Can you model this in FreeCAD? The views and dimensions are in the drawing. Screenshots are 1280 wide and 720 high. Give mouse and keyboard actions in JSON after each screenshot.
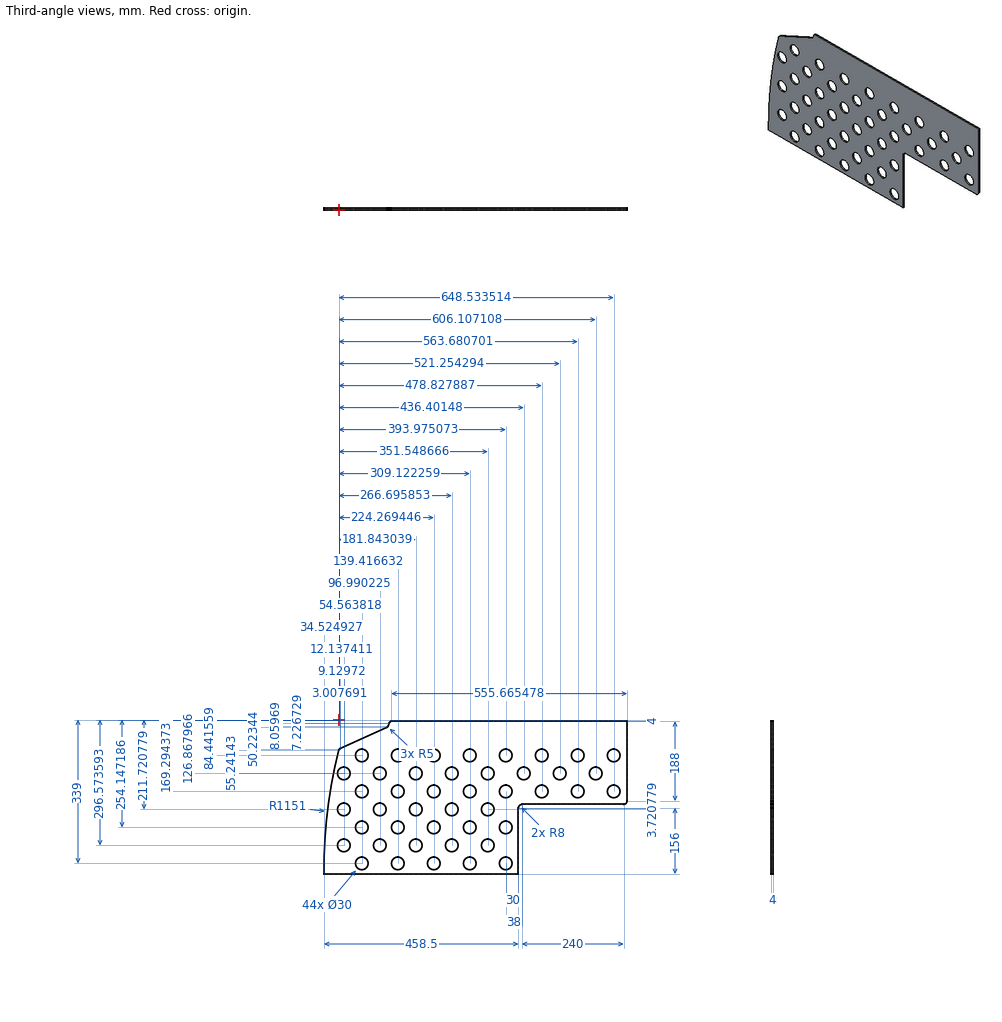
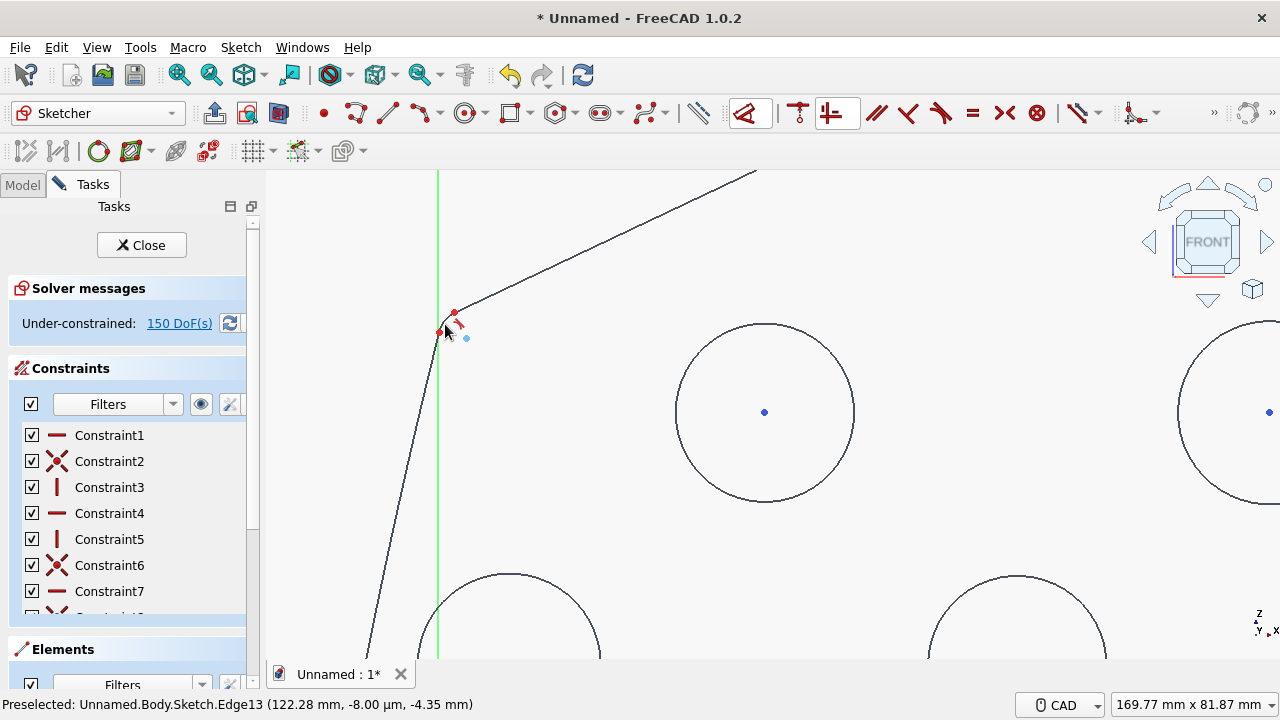
{"action": "left_click", "coordinate": [439, 326]}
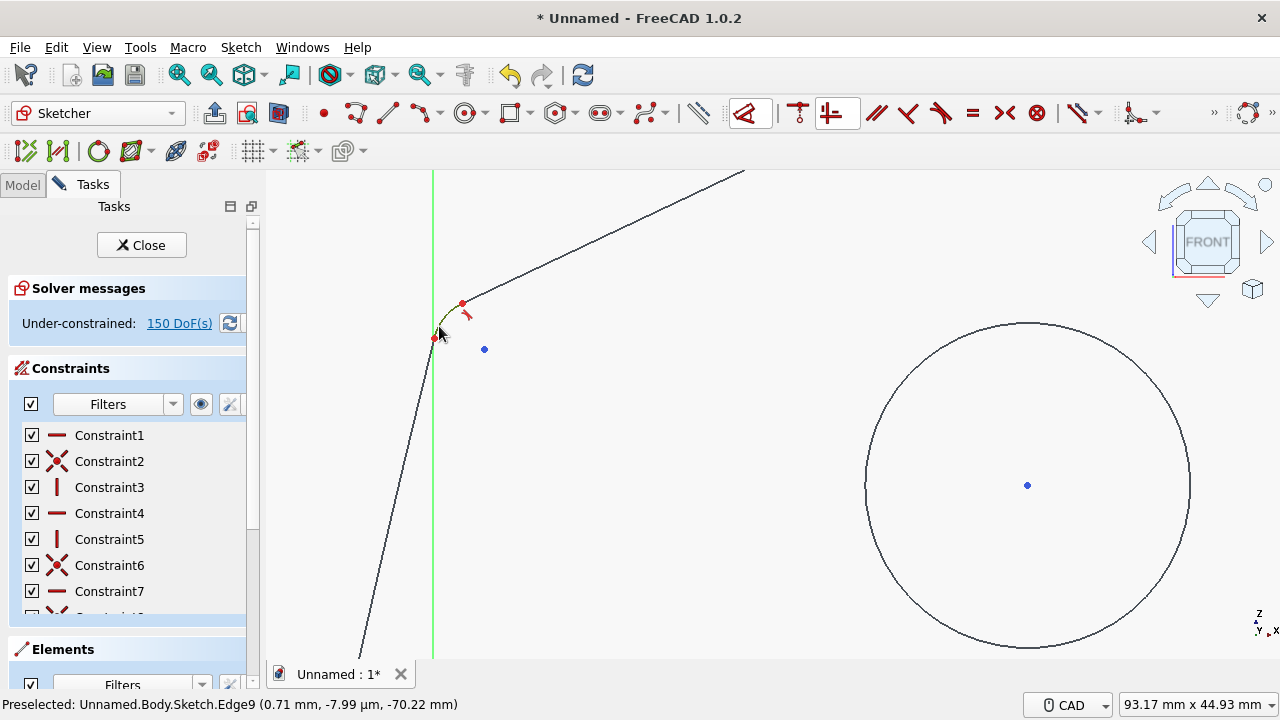
{"action": "scroll", "coordinate": [445, 324], "scroll_direction": "down", "scroll_amount": 13}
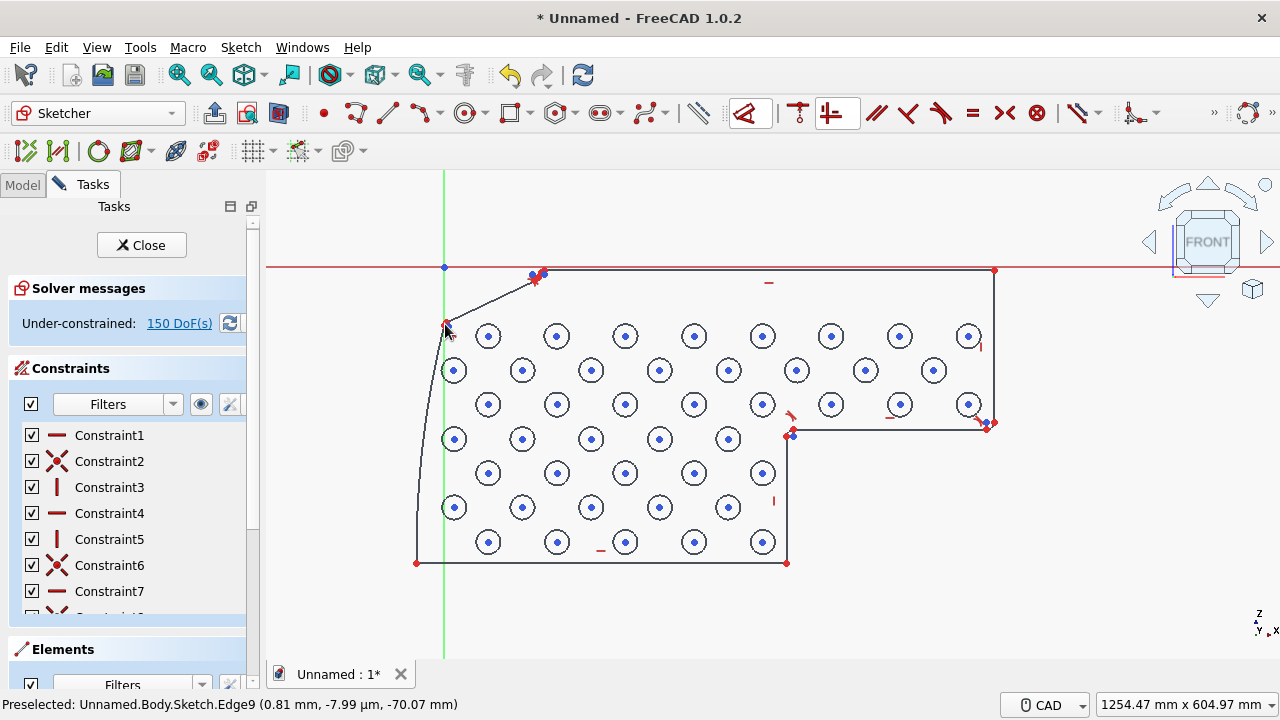
{"action": "left_click", "coordinate": [430, 396]}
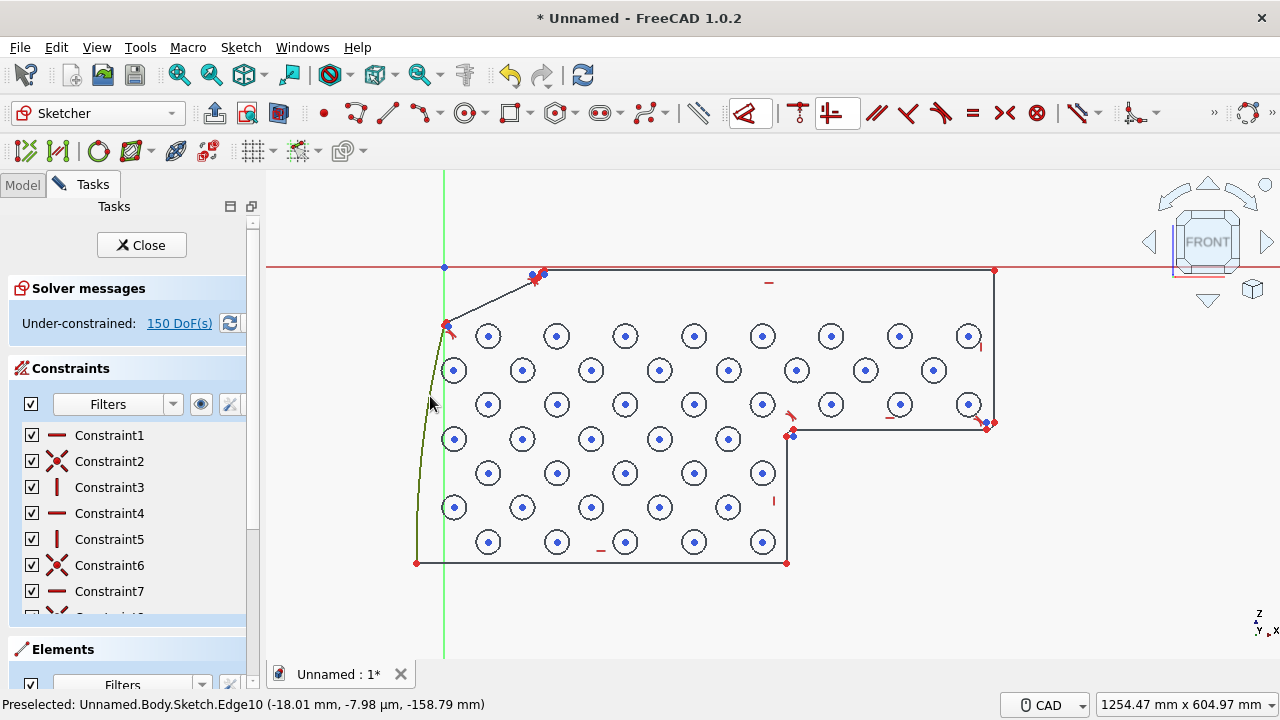
{"action": "left_click", "coordinate": [942, 114]}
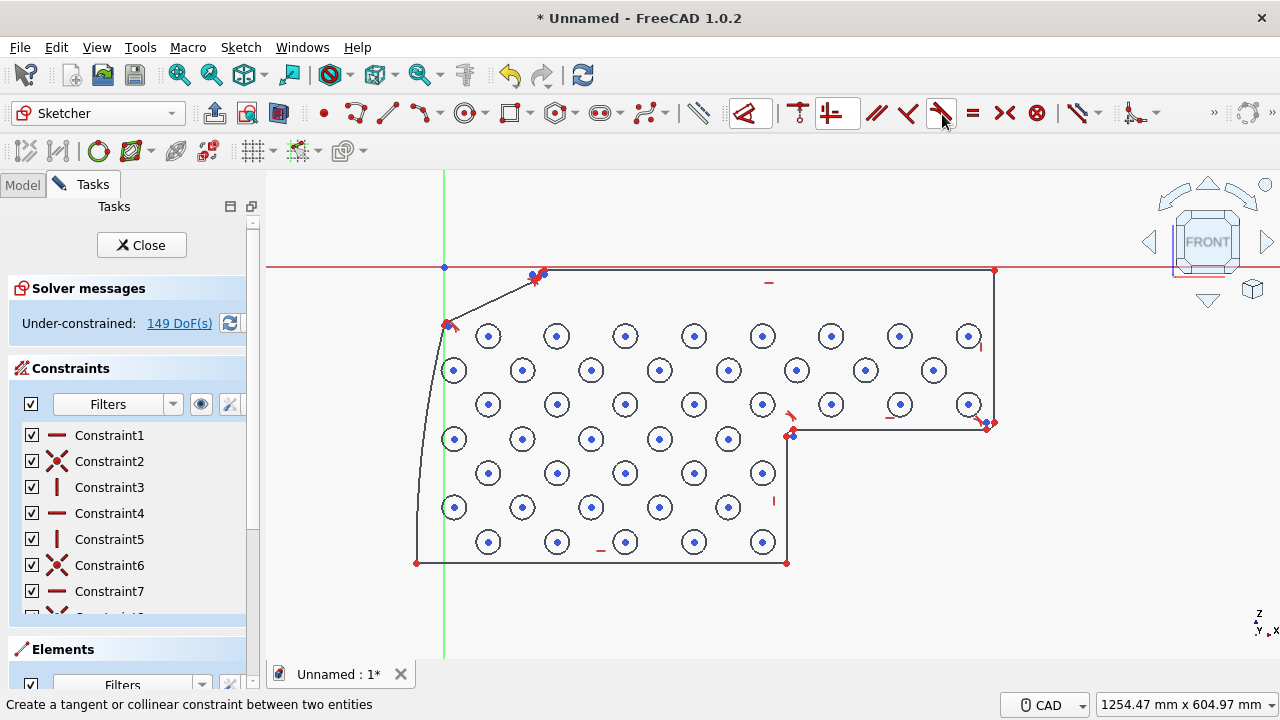
{"action": "scroll", "coordinate": [537, 280], "scroll_direction": "up", "scroll_amount": 10}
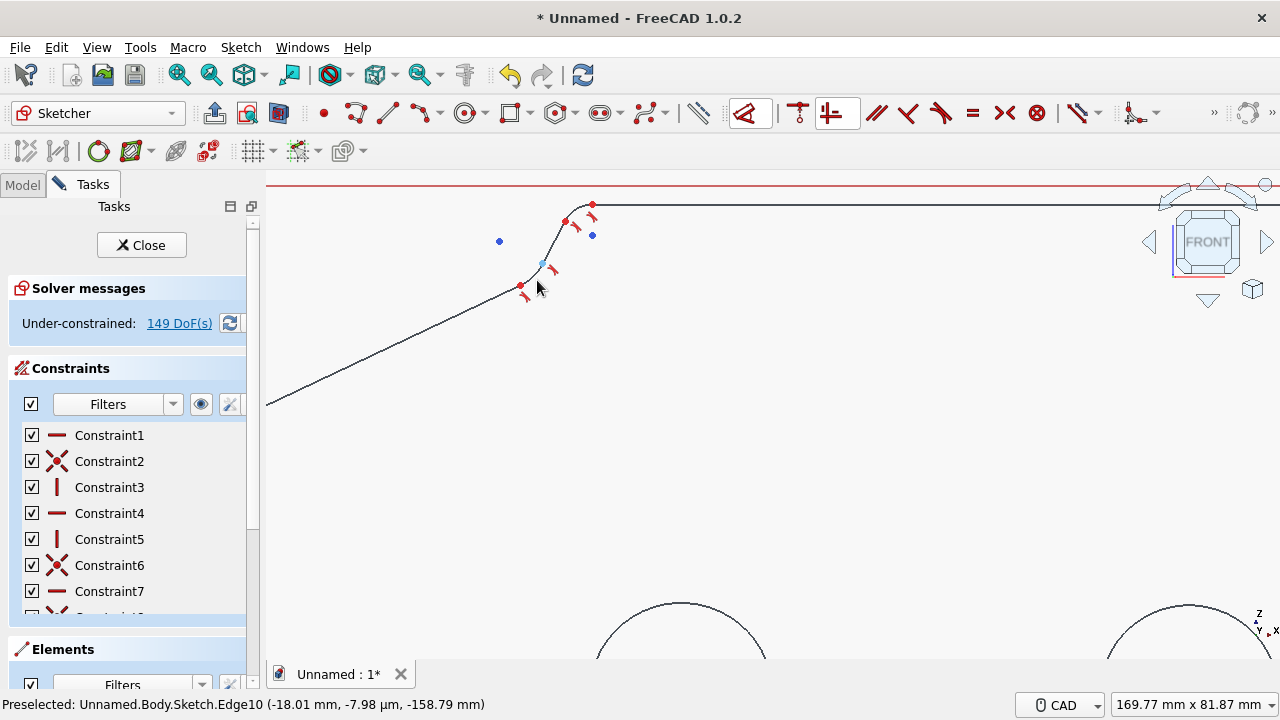
{"action": "left_click", "coordinate": [533, 276]}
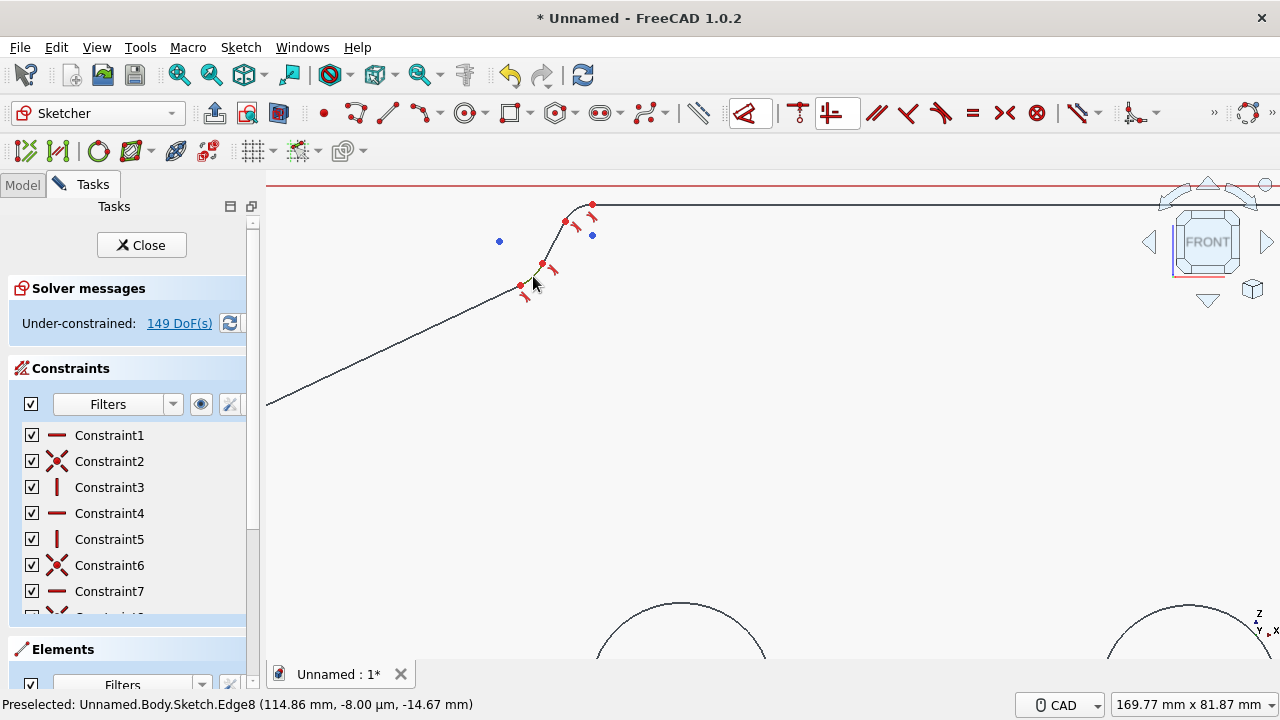
{"action": "scroll", "coordinate": [537, 280], "scroll_direction": "down", "scroll_amount": 10}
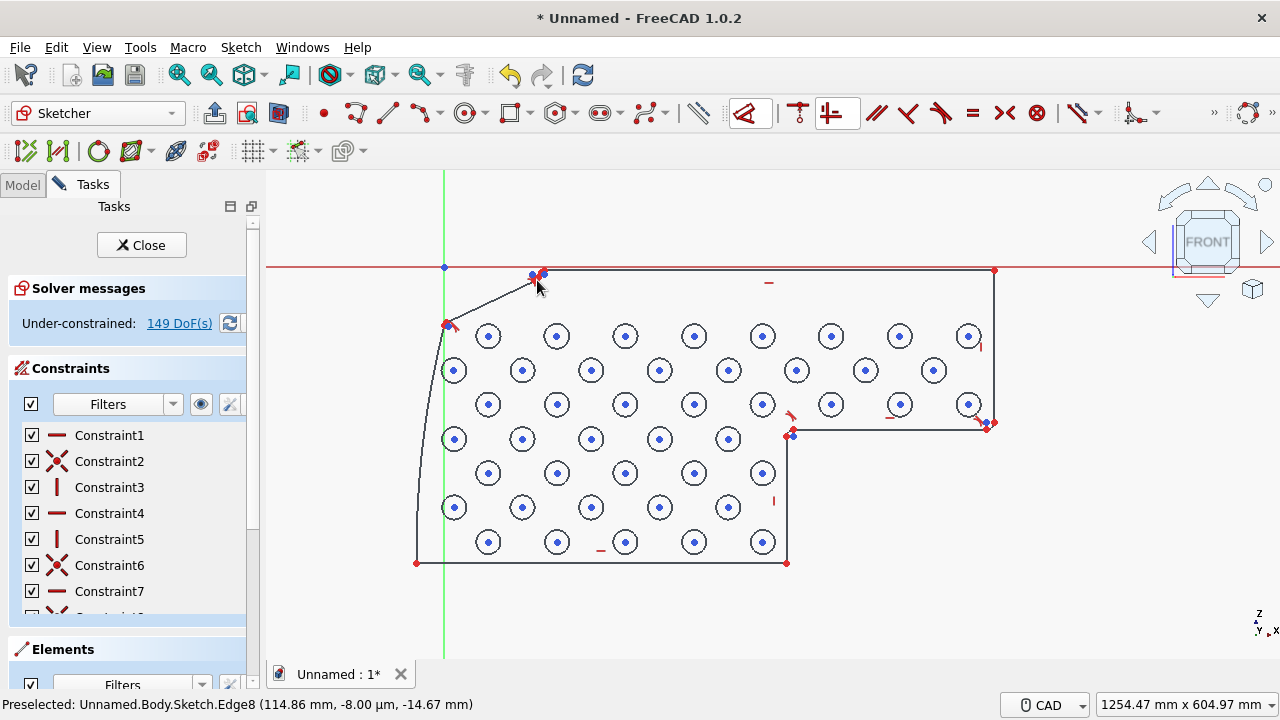
{"action": "scroll", "coordinate": [445, 324], "scroll_direction": "up", "scroll_amount": 14}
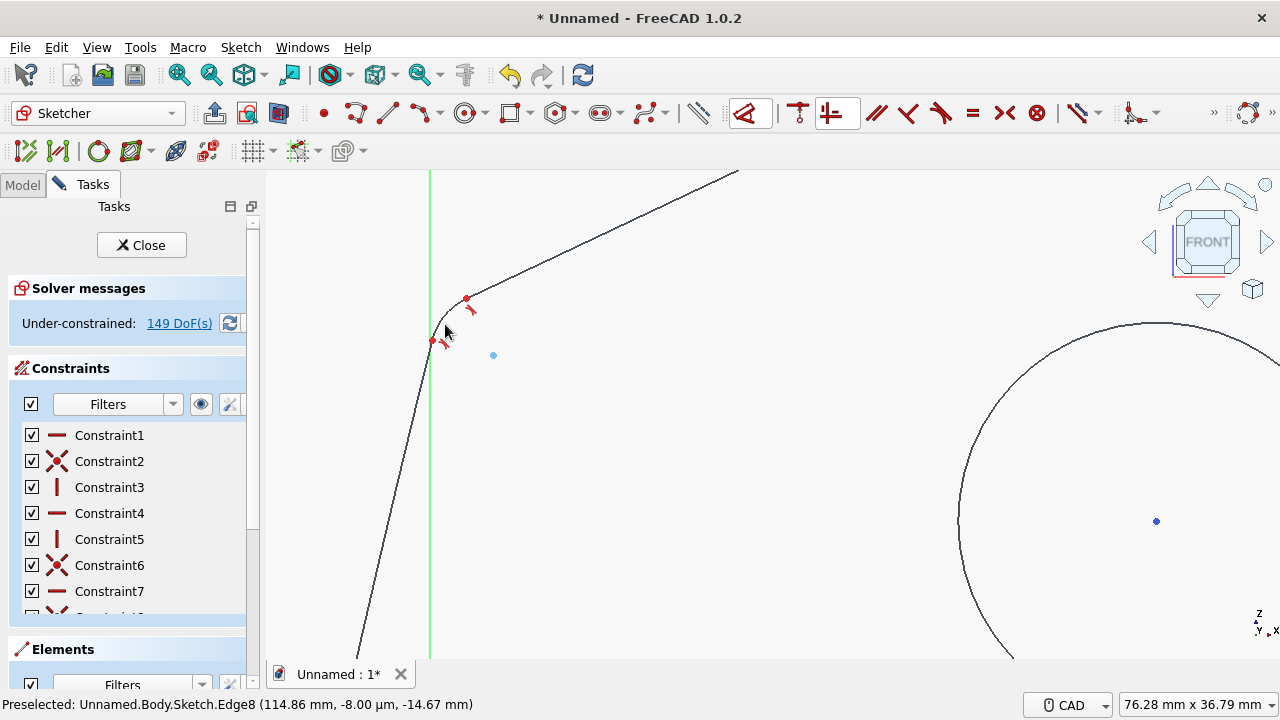
{"action": "left_click", "coordinate": [438, 325]}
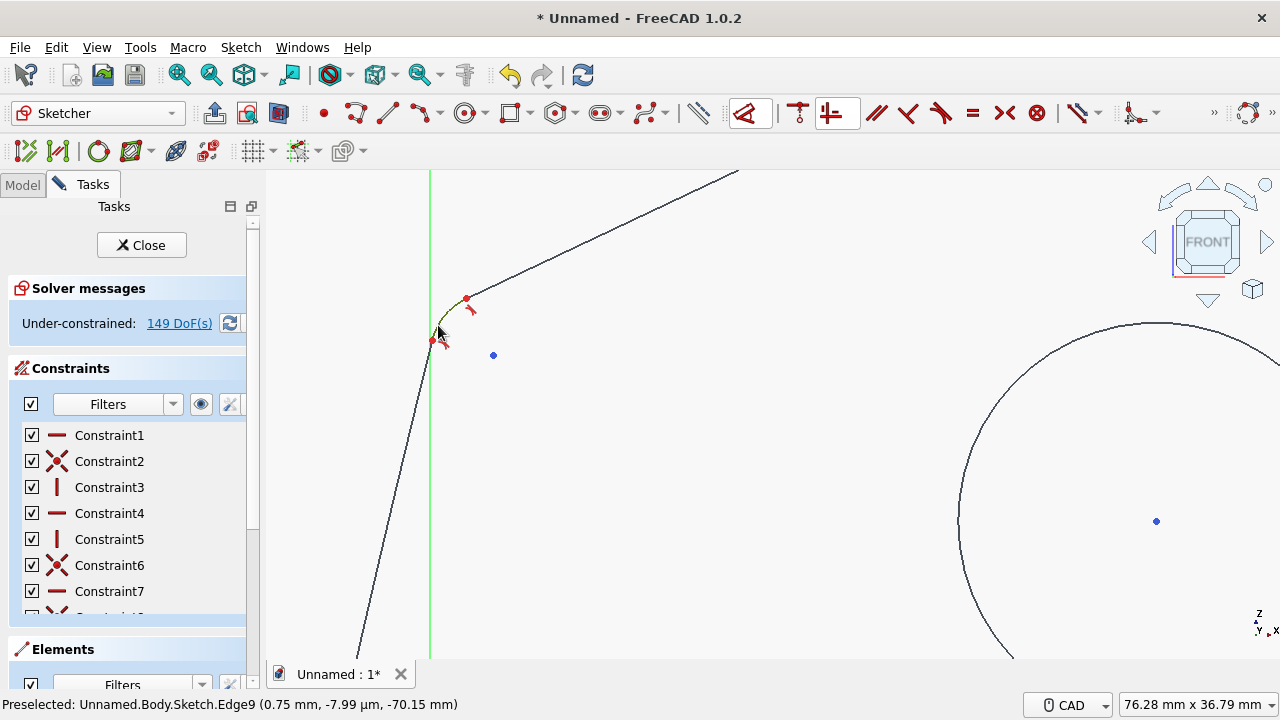
{"action": "scroll", "coordinate": [445, 324], "scroll_direction": "down", "scroll_amount": 14}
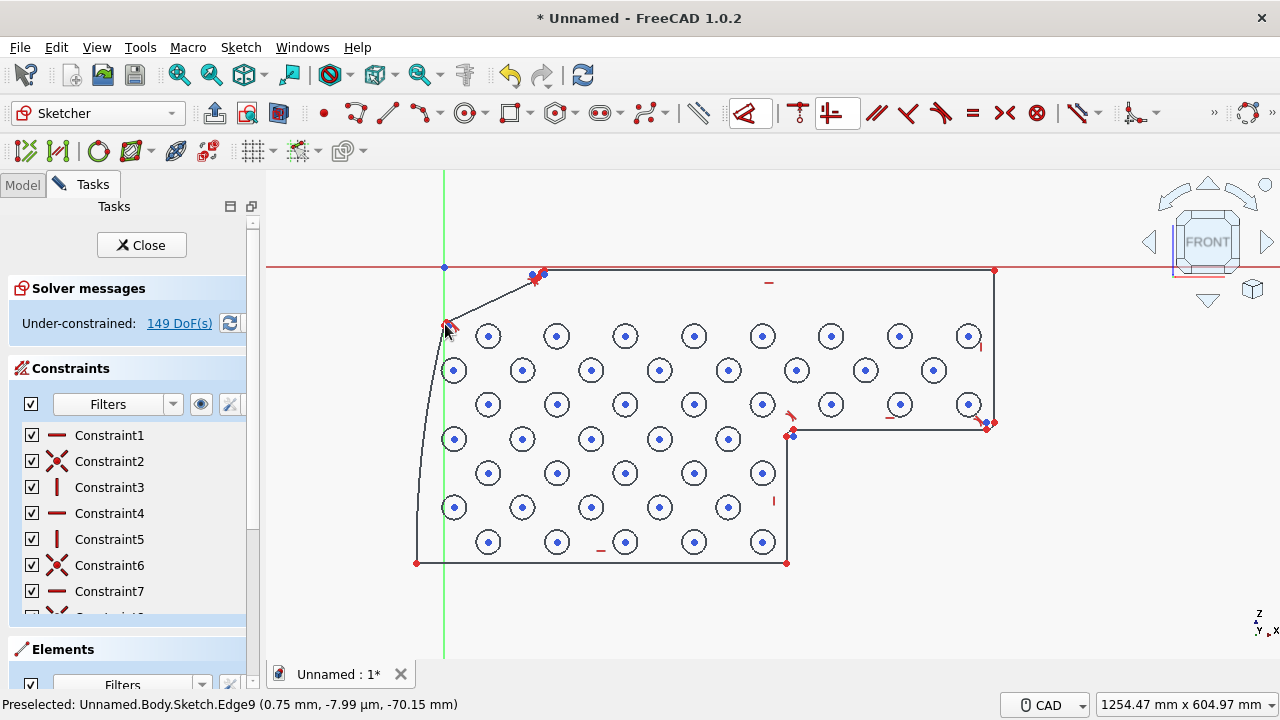
{"action": "scroll", "coordinate": [543, 270], "scroll_direction": "up", "scroll_amount": 12}